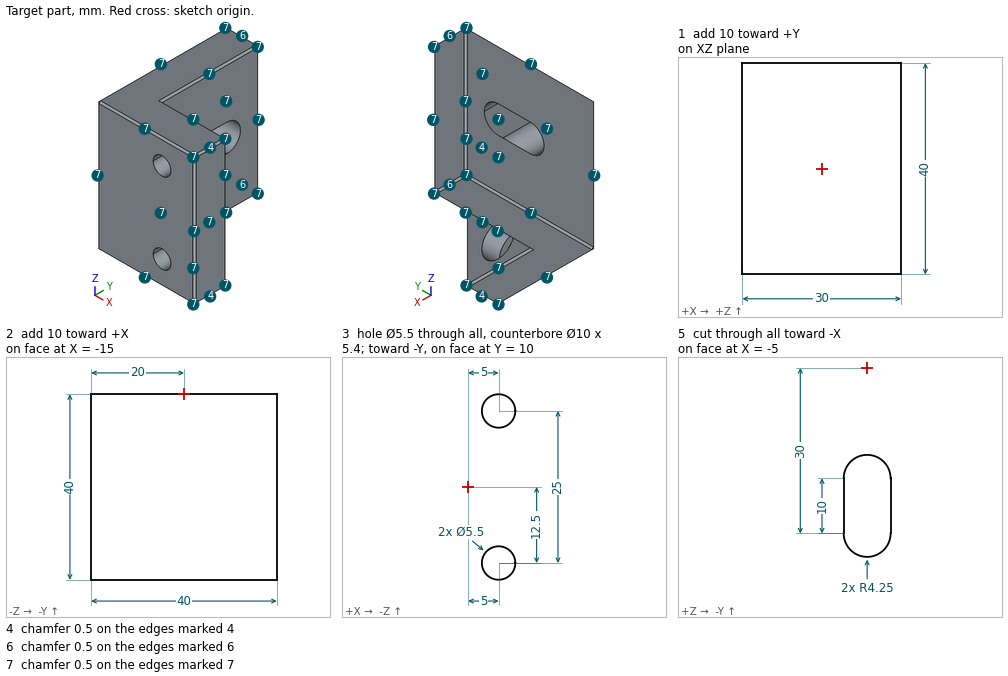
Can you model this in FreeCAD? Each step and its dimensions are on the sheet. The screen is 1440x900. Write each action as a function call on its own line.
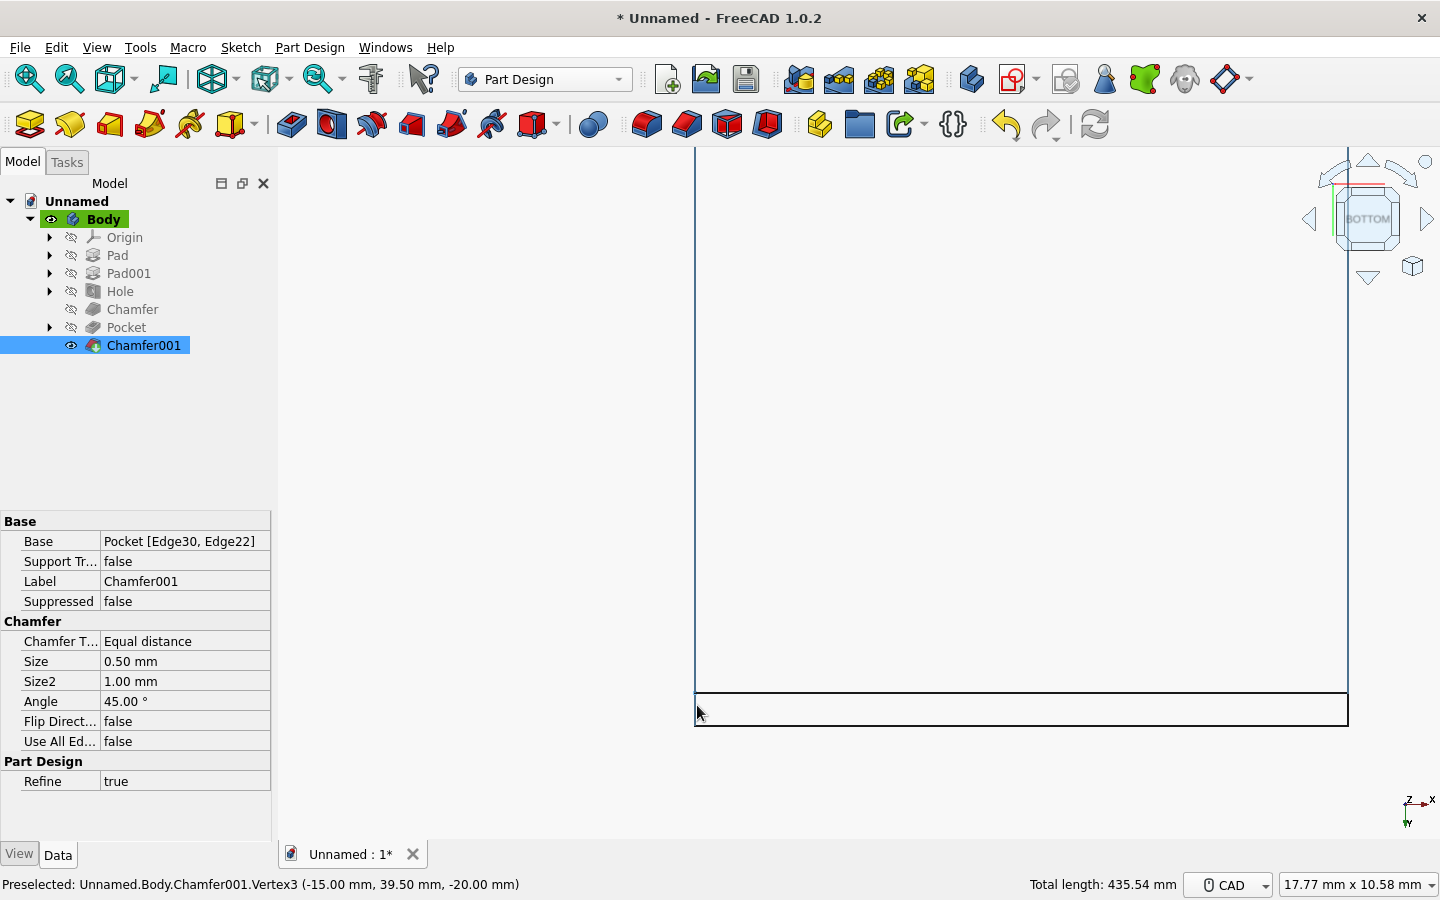
click(1348, 709, ctrl)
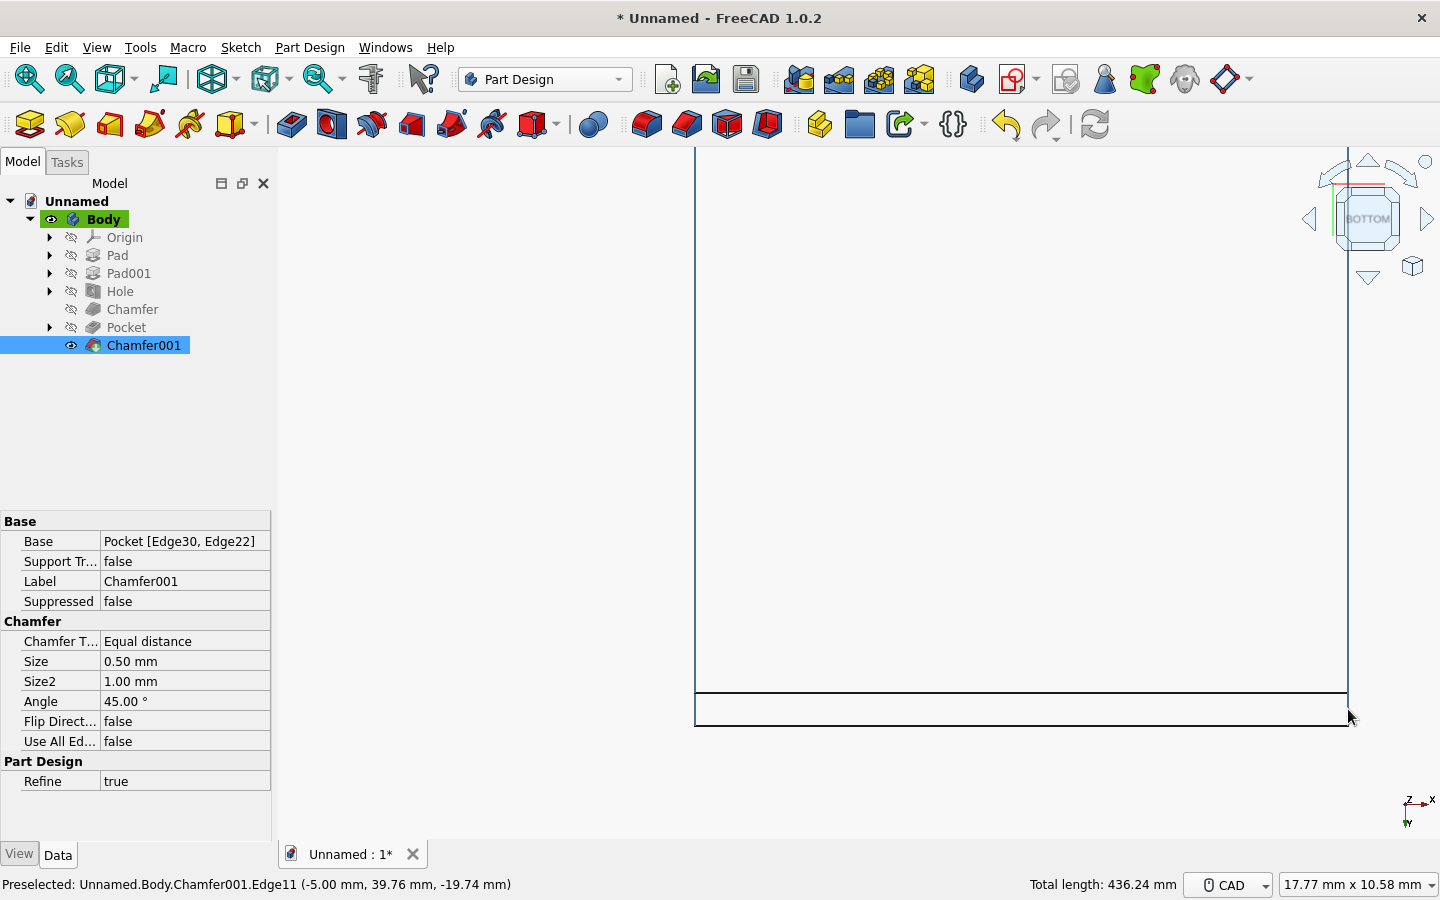
click(30, 80)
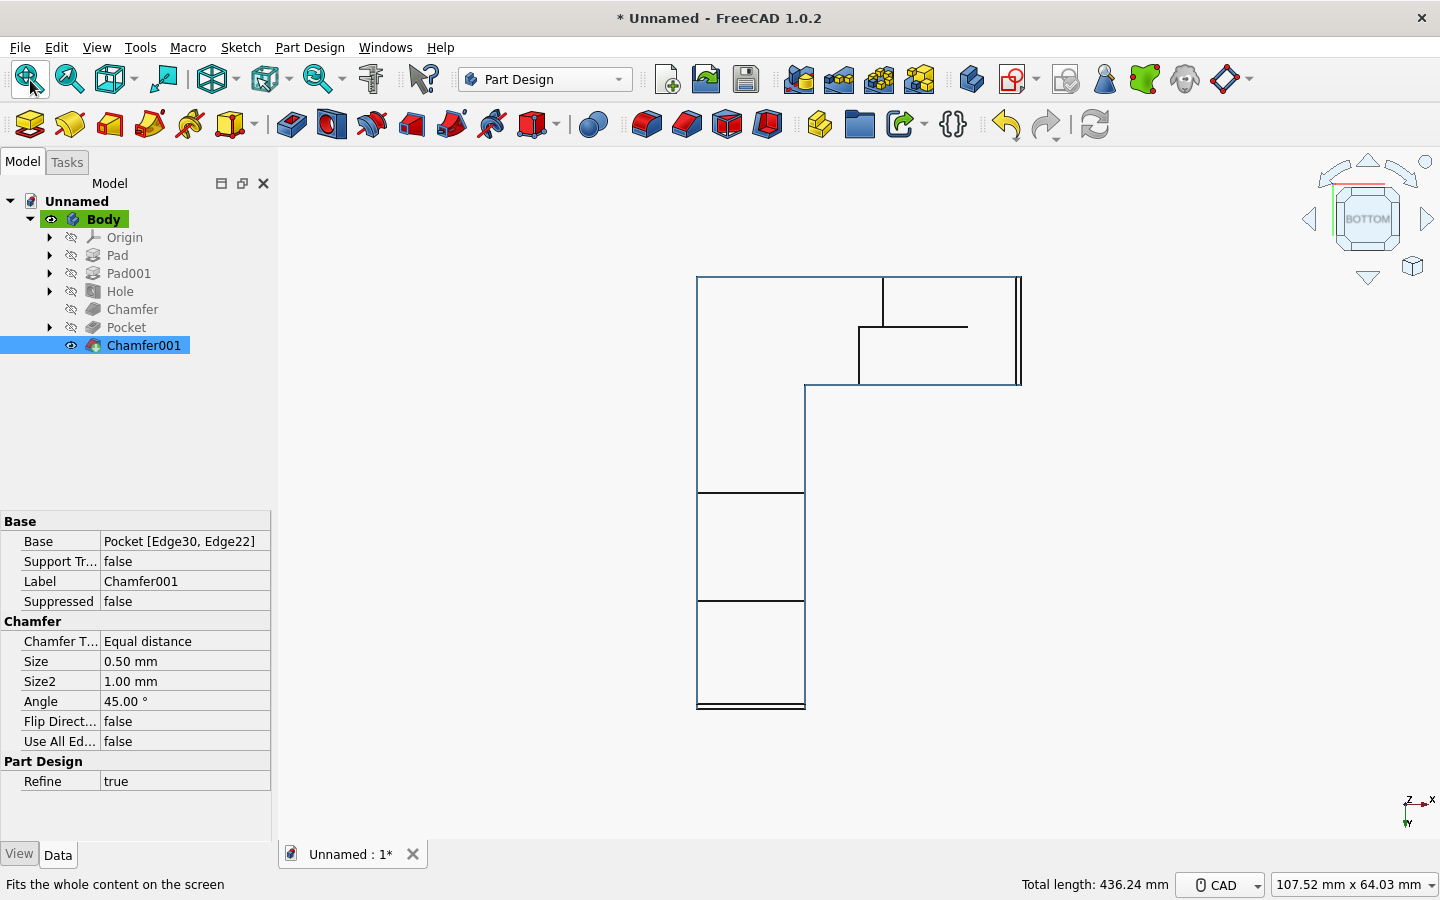
key(4)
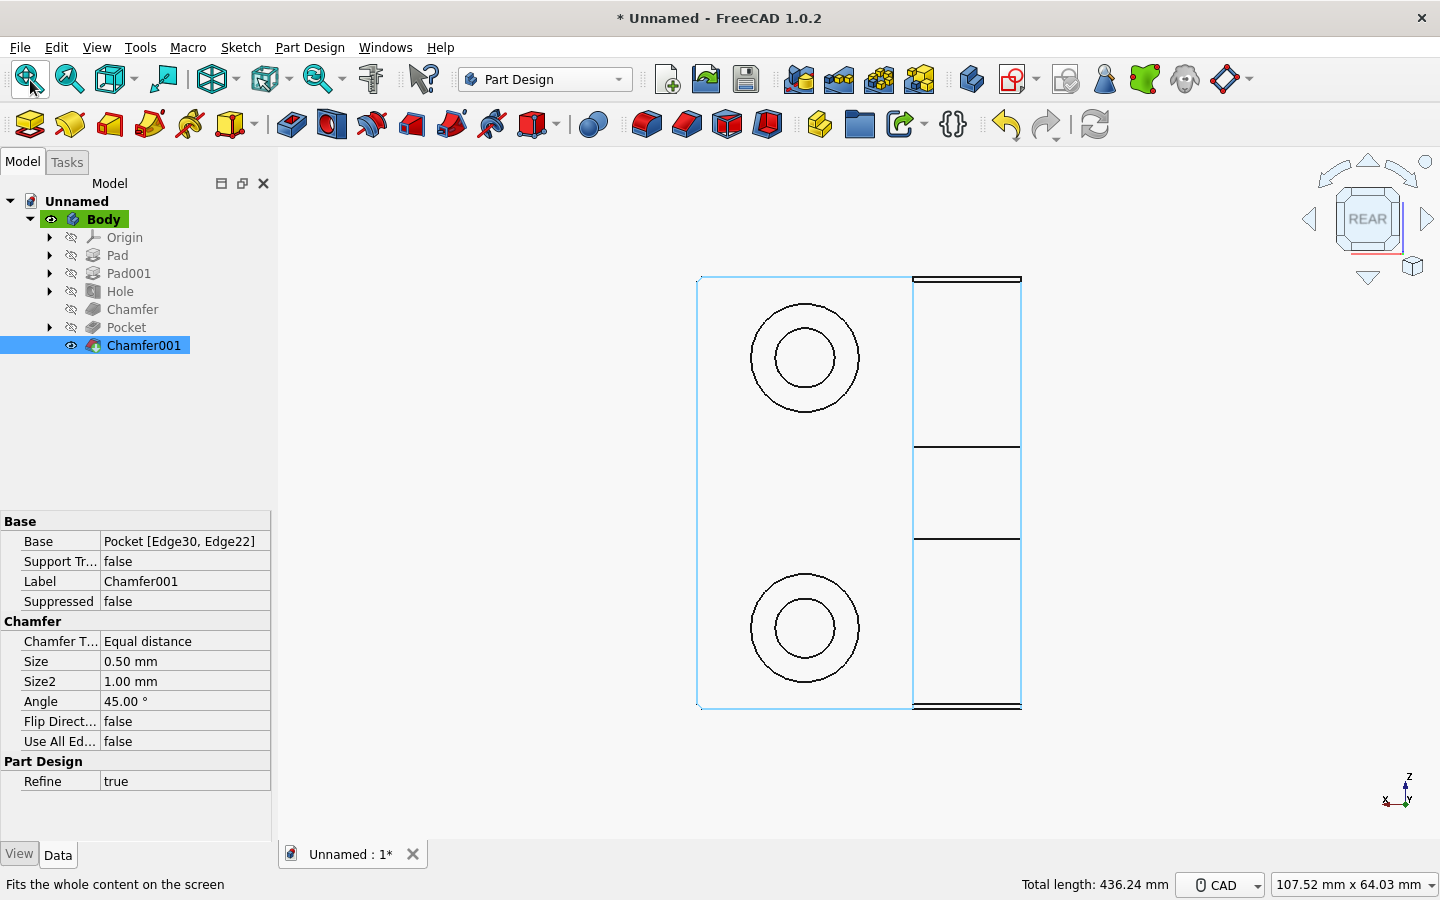
scroll(1021, 279, up, 9)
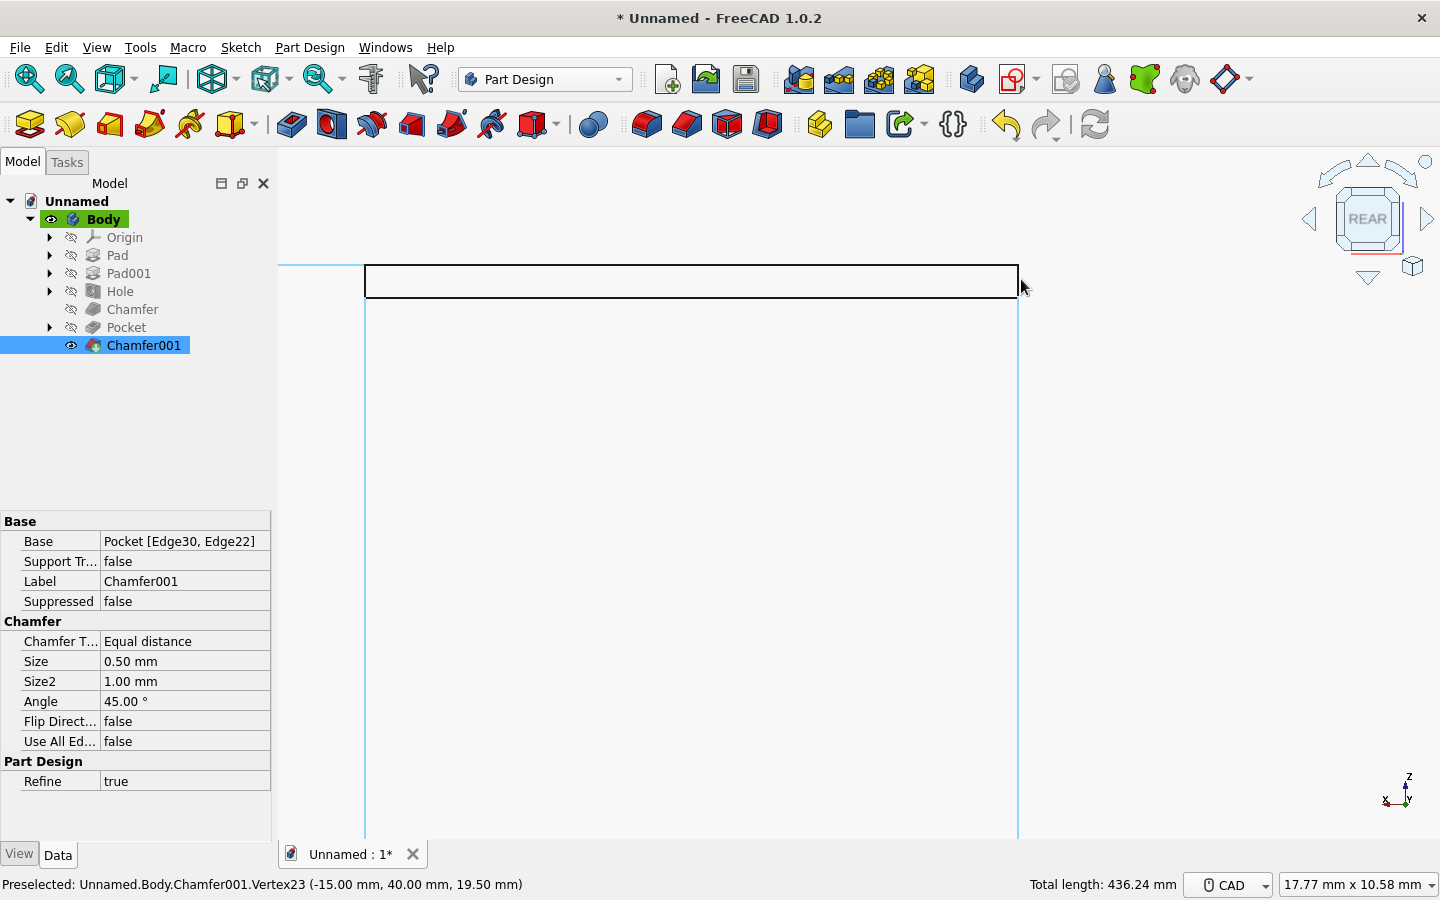
click(1018, 280, ctrl)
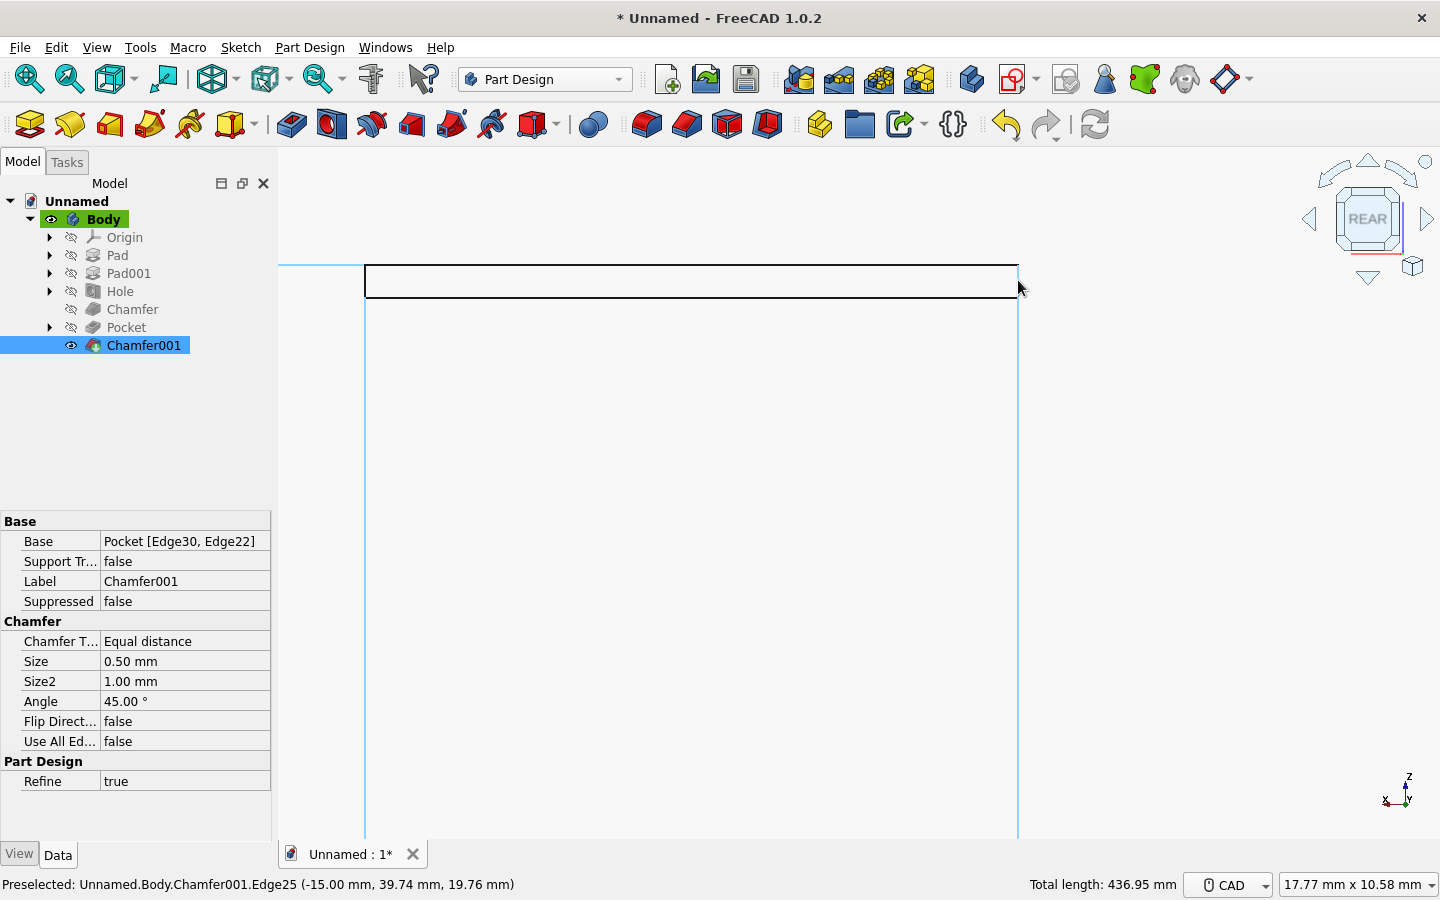
click(365, 280, ctrl)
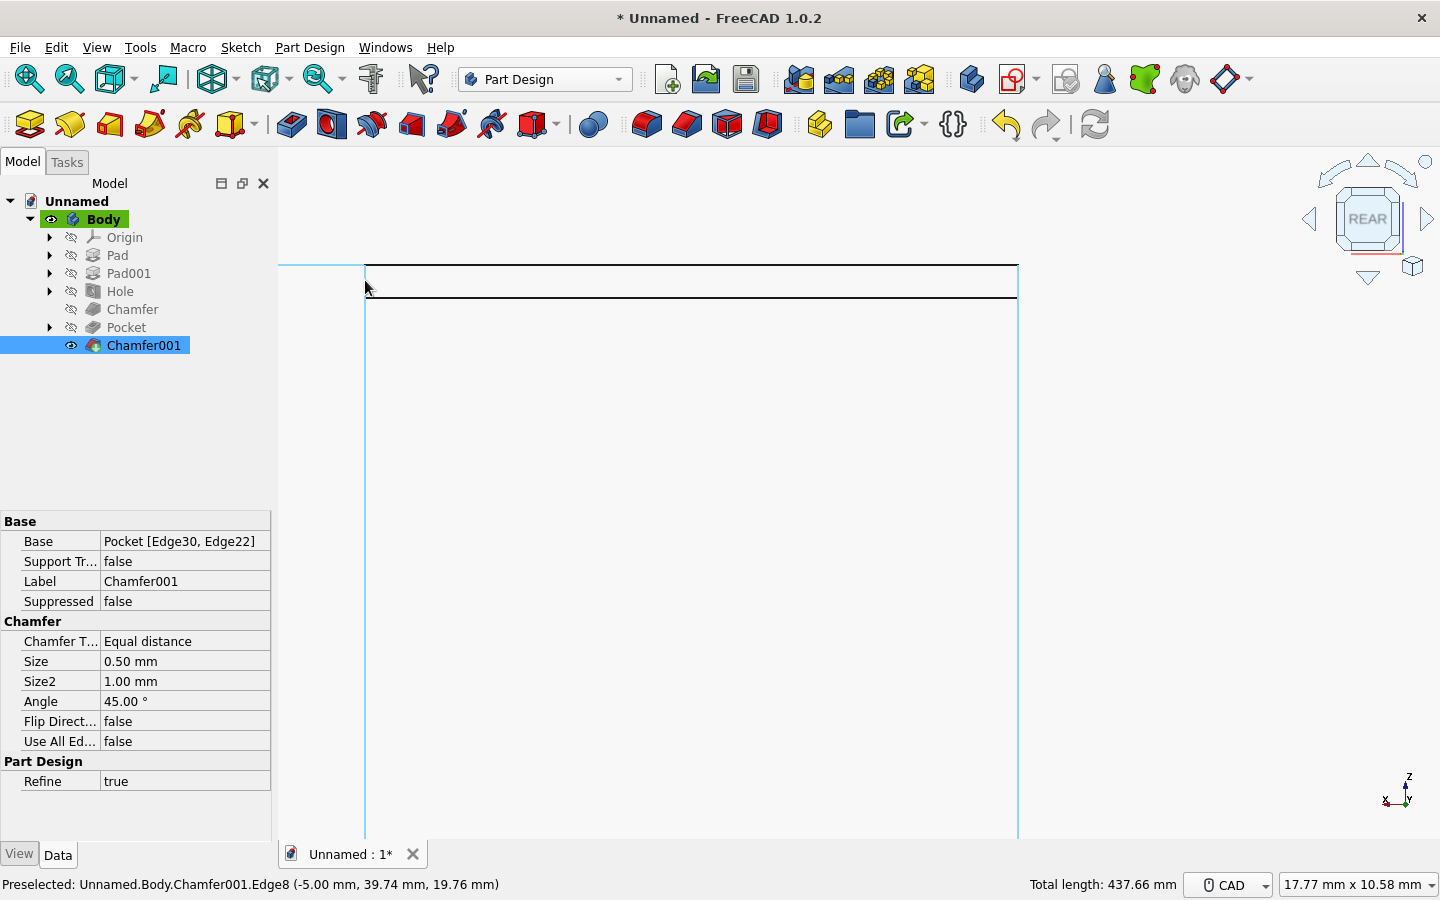
key(v)
key(1)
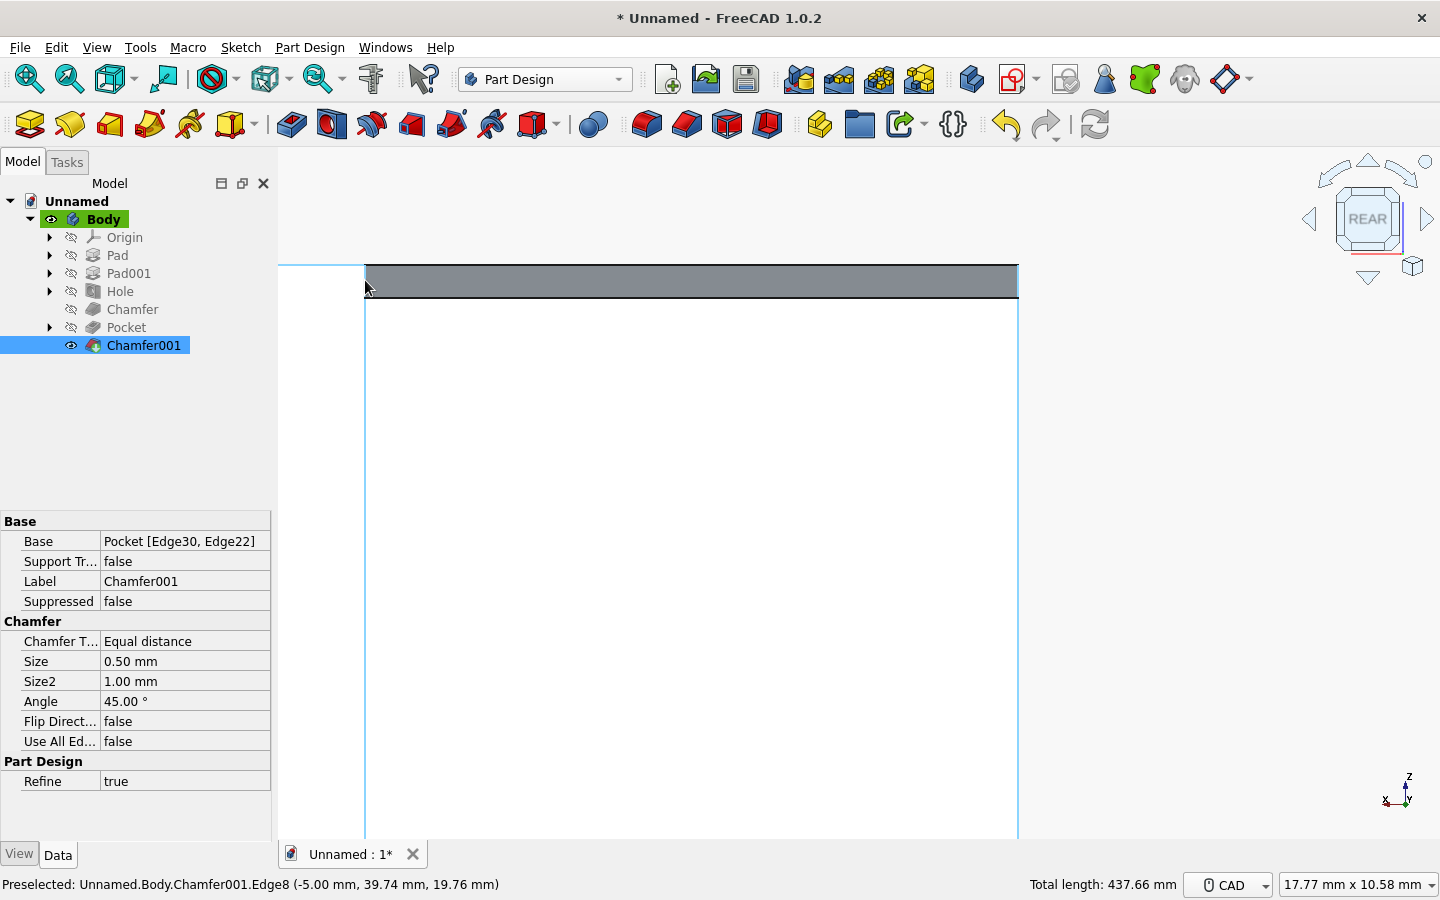
click(688, 124)